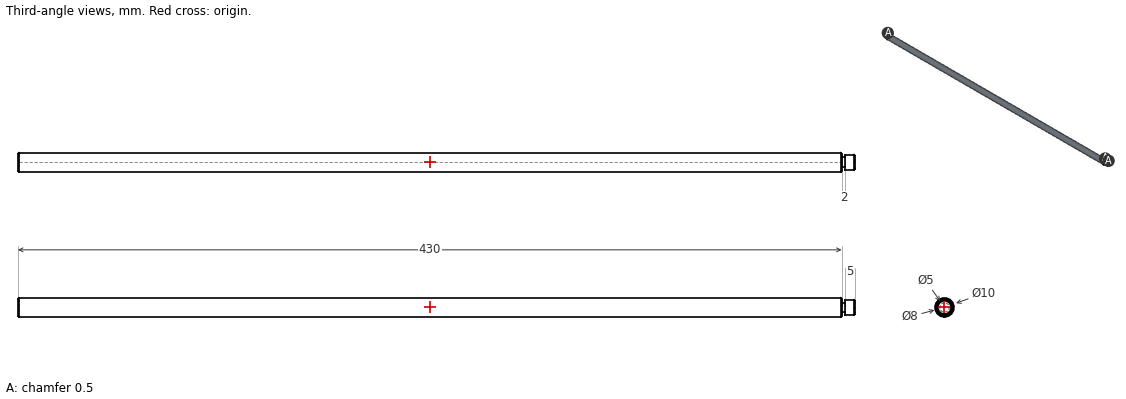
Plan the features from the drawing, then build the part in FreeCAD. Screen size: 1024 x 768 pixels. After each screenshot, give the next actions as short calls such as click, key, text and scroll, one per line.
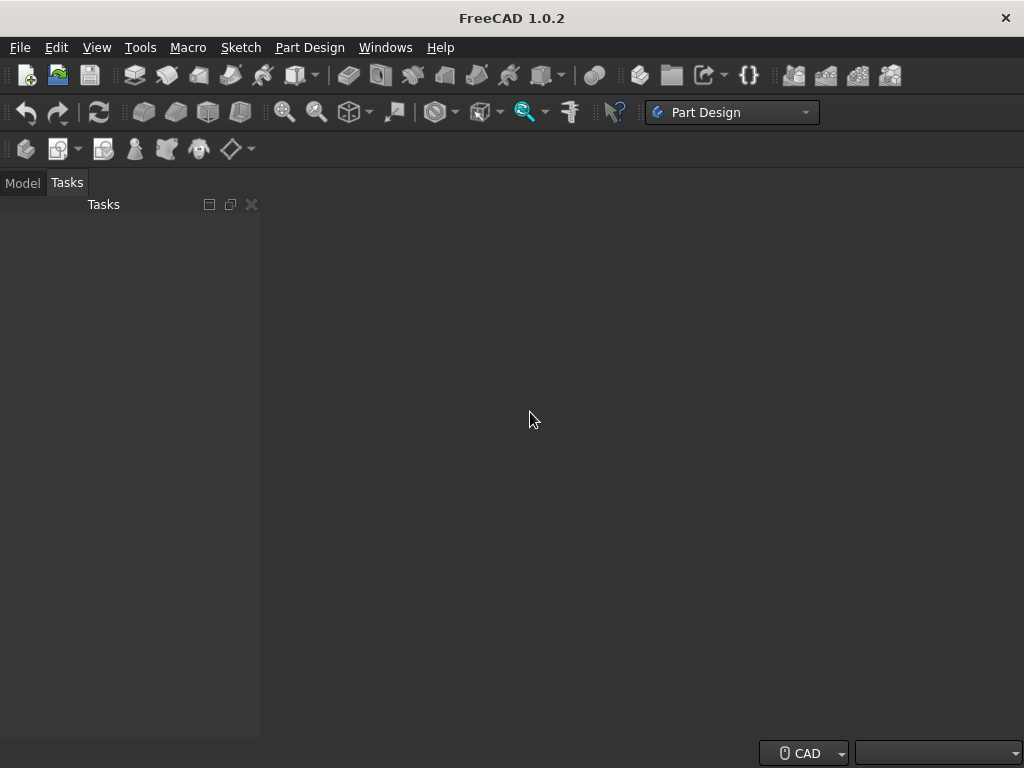
click(26, 76)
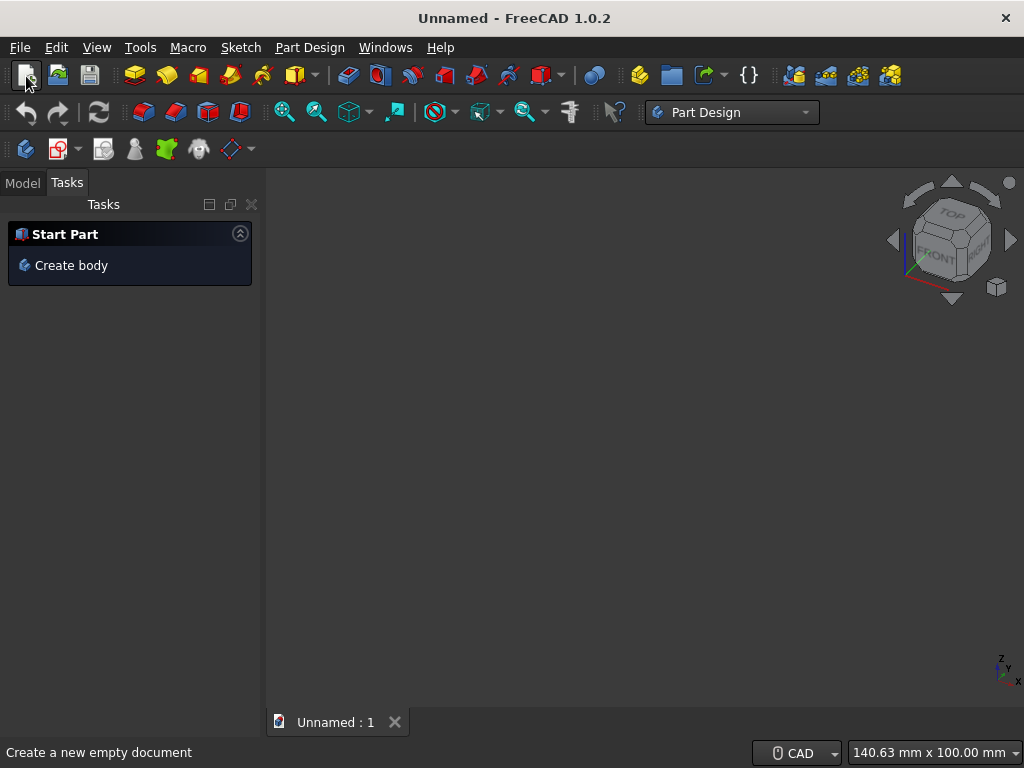
click(58, 150)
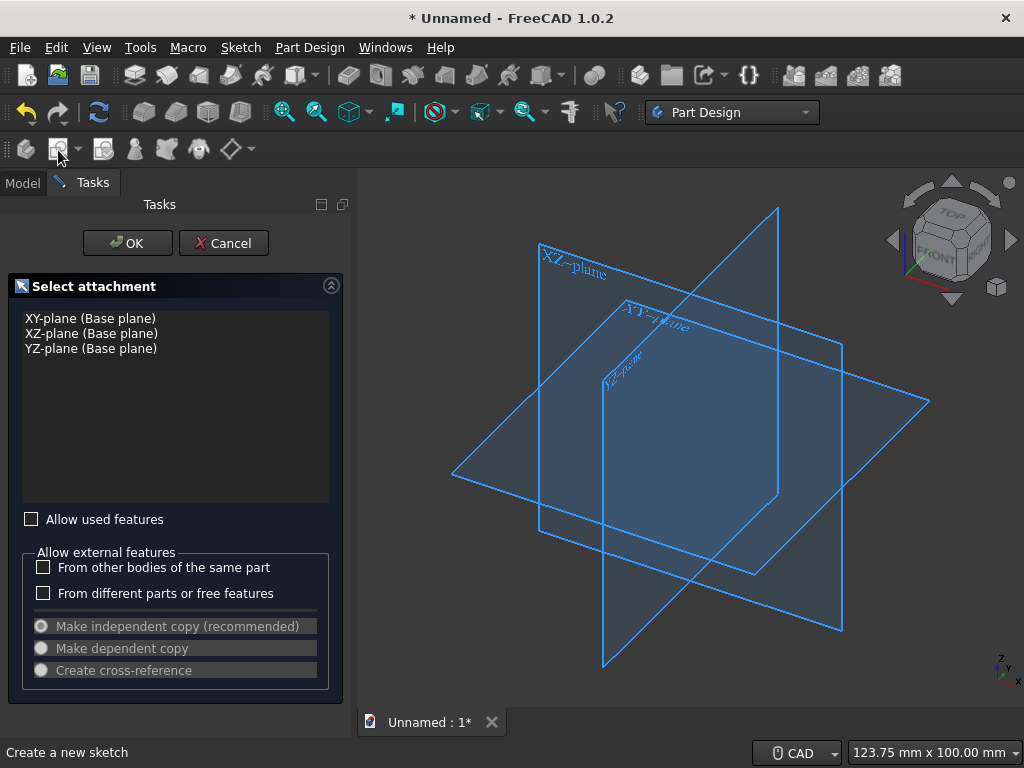
click(82, 348)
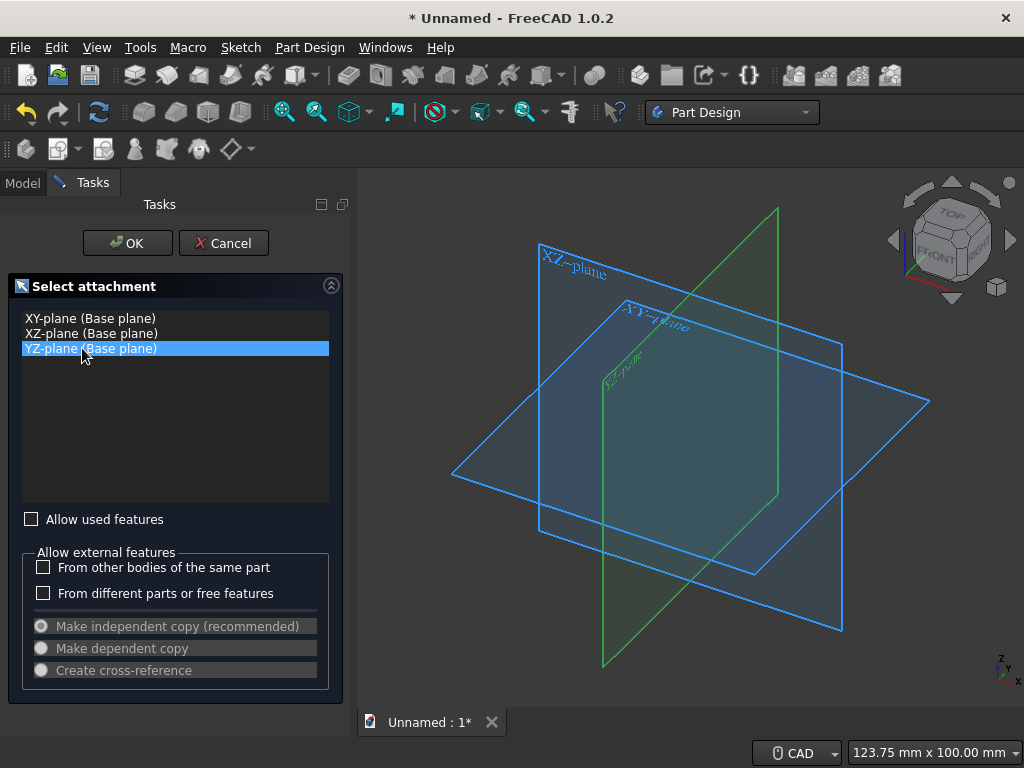
click(128, 243)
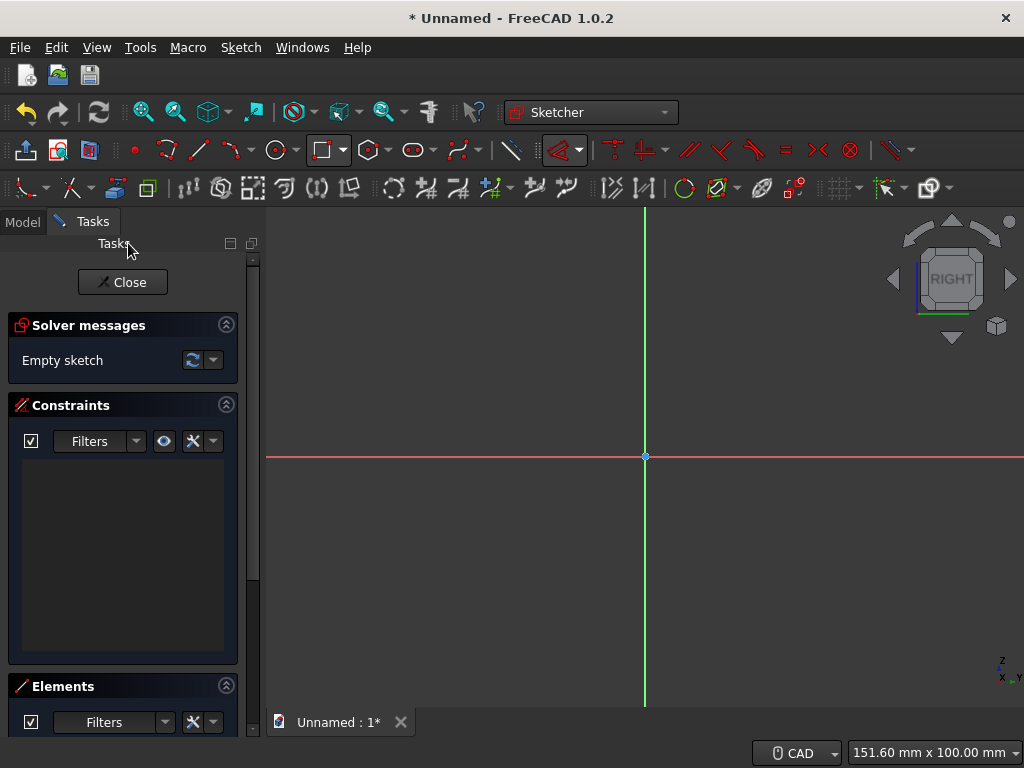
scroll(659, 457, up, 9)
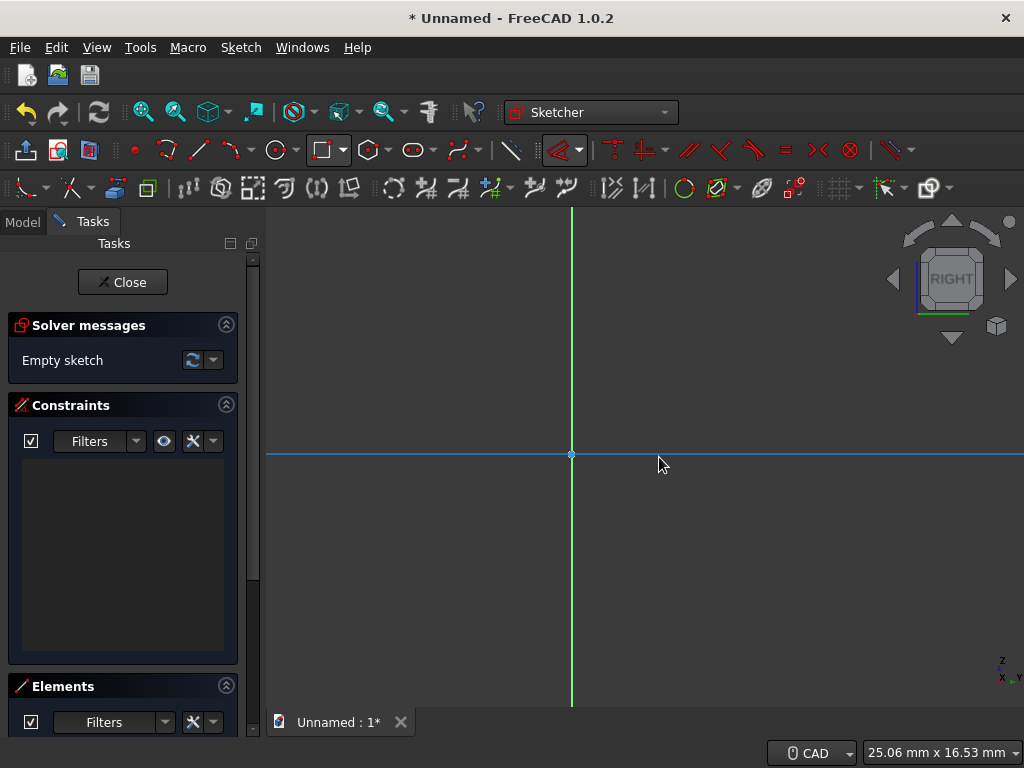
click(276, 150)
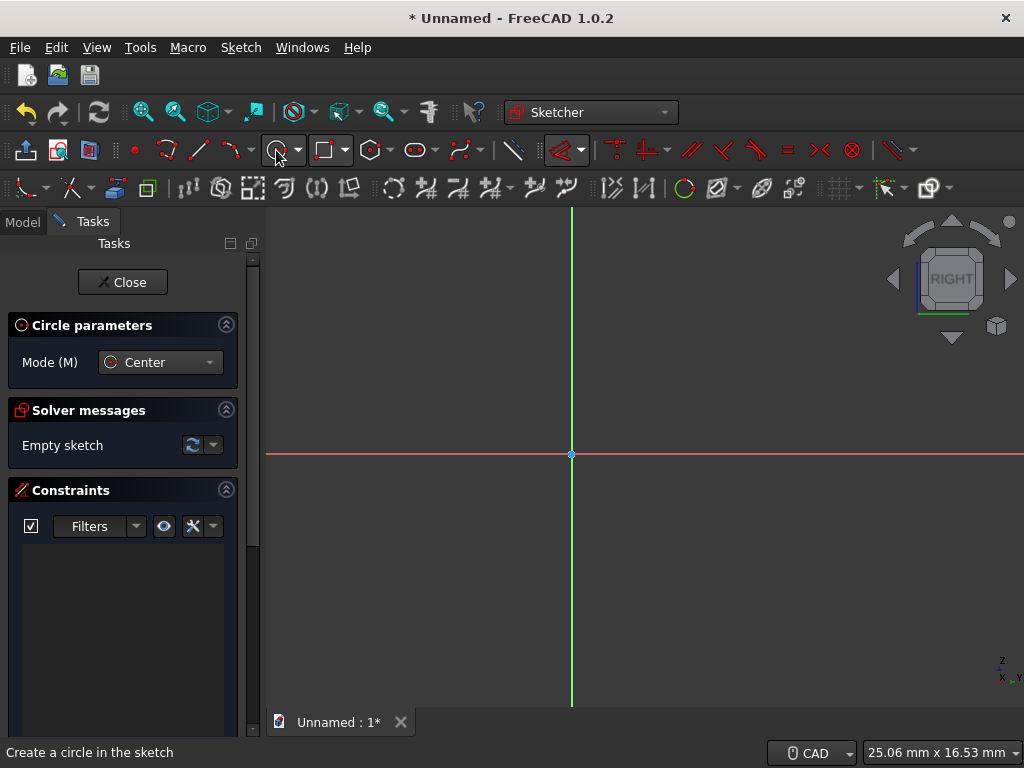
click(572, 454)
move(679, 348)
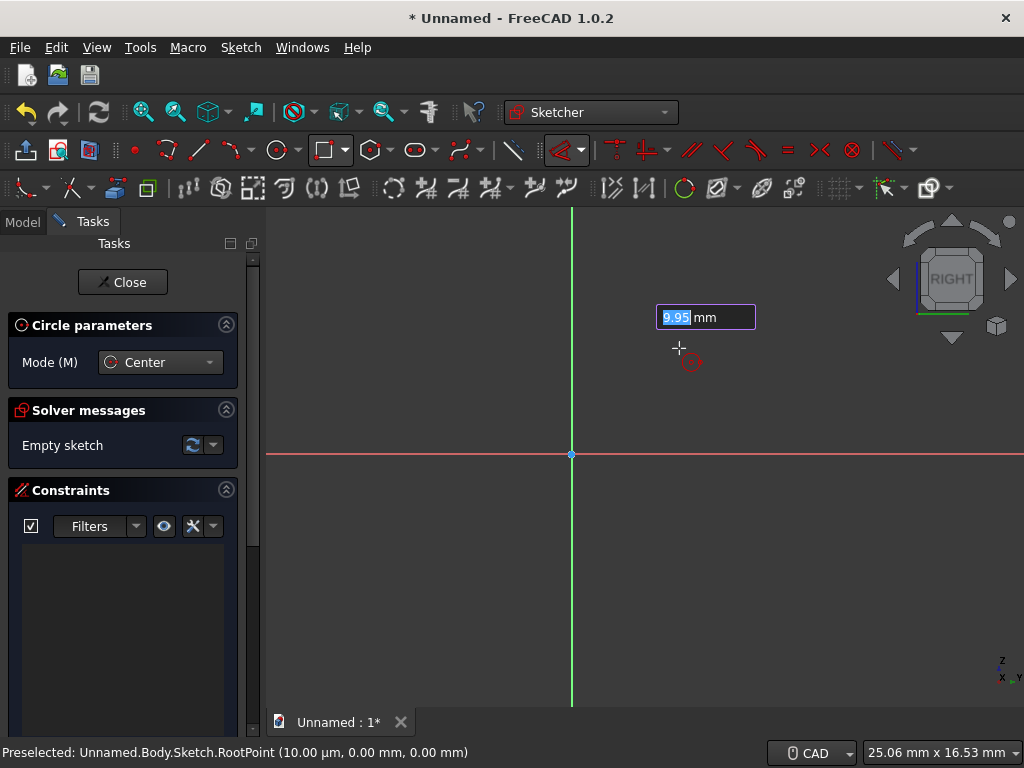
text(10)
key(Return)
key(Escape)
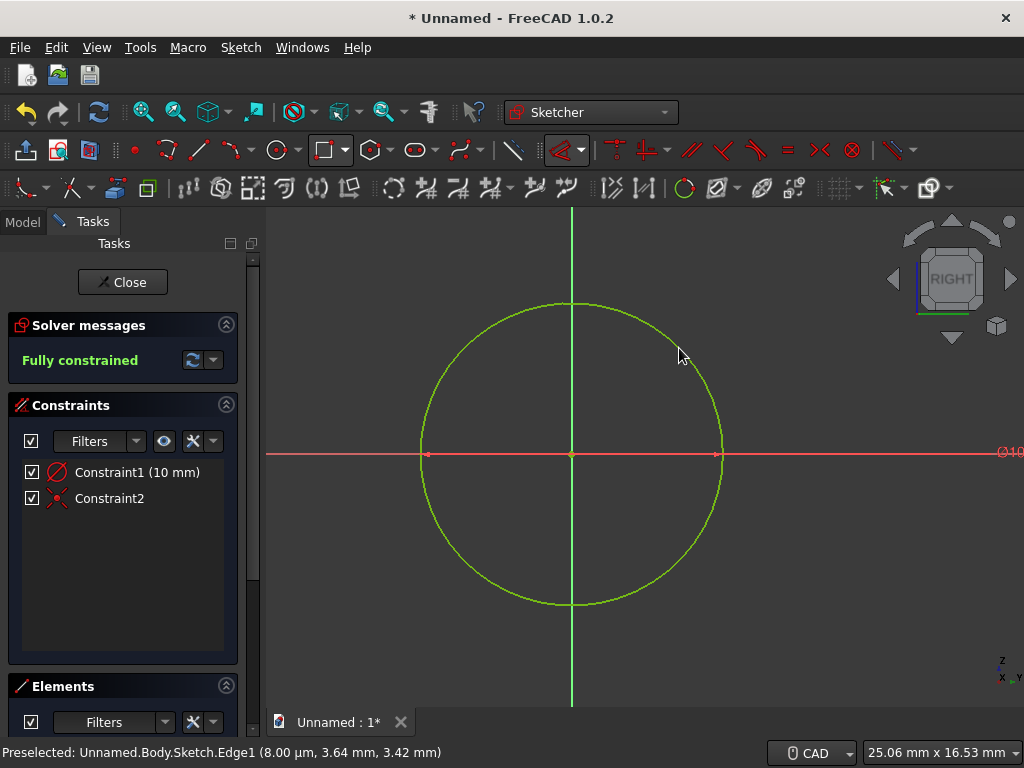
click(123, 282)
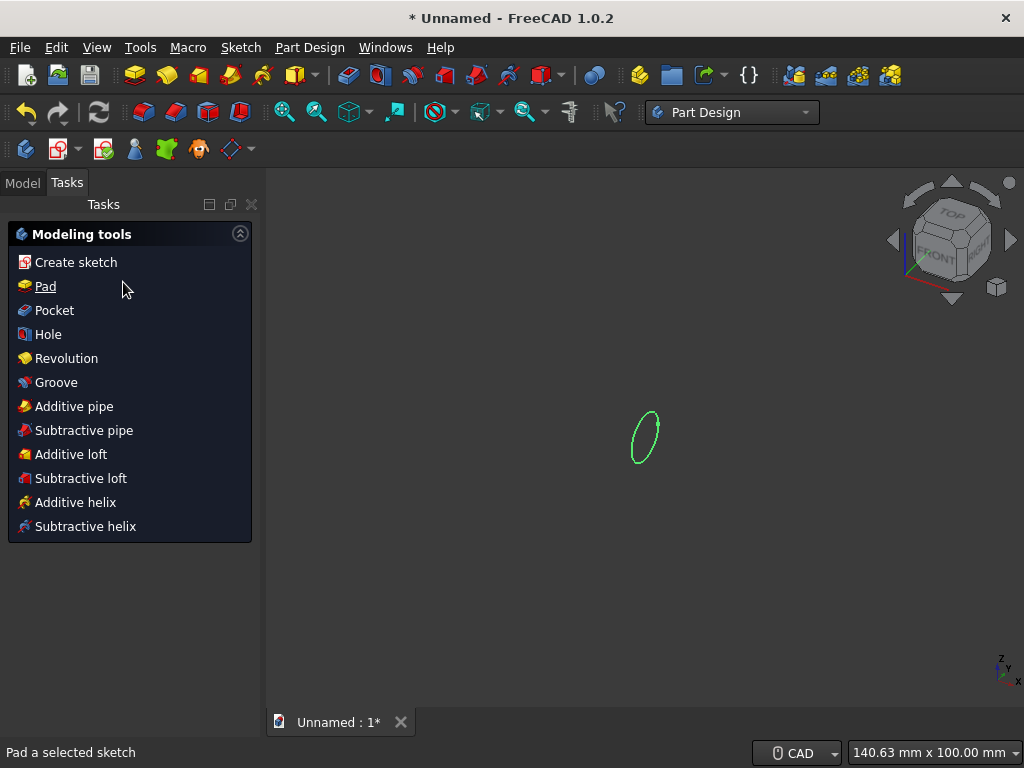
click(136, 76)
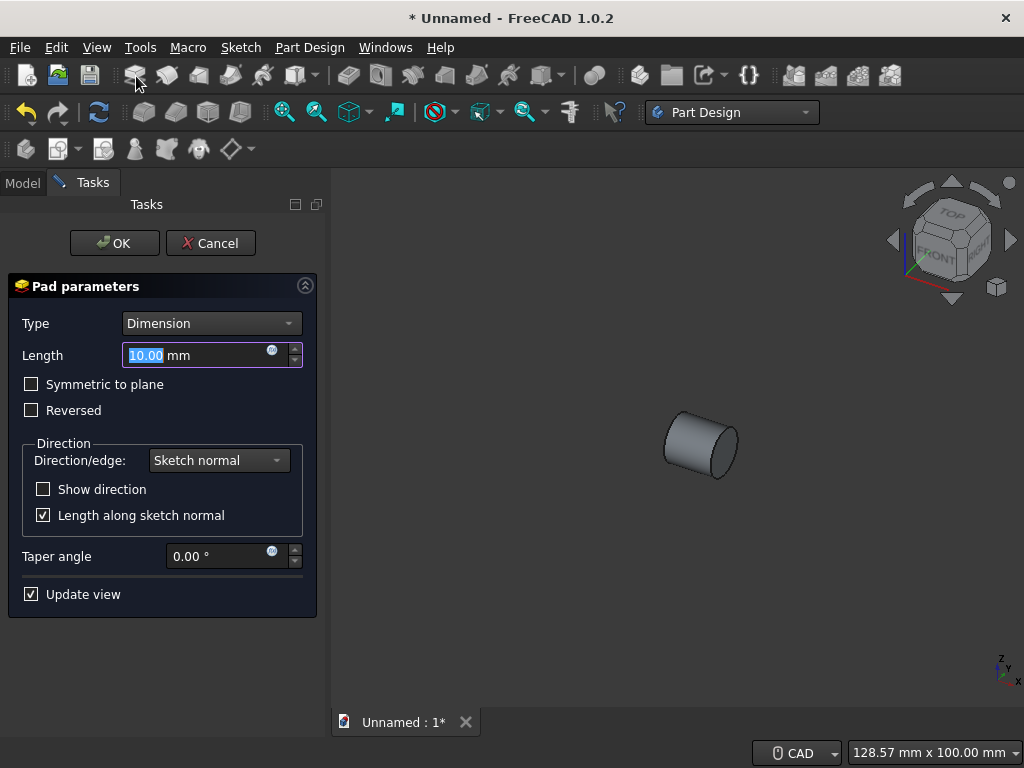
text(430)
key(Tab)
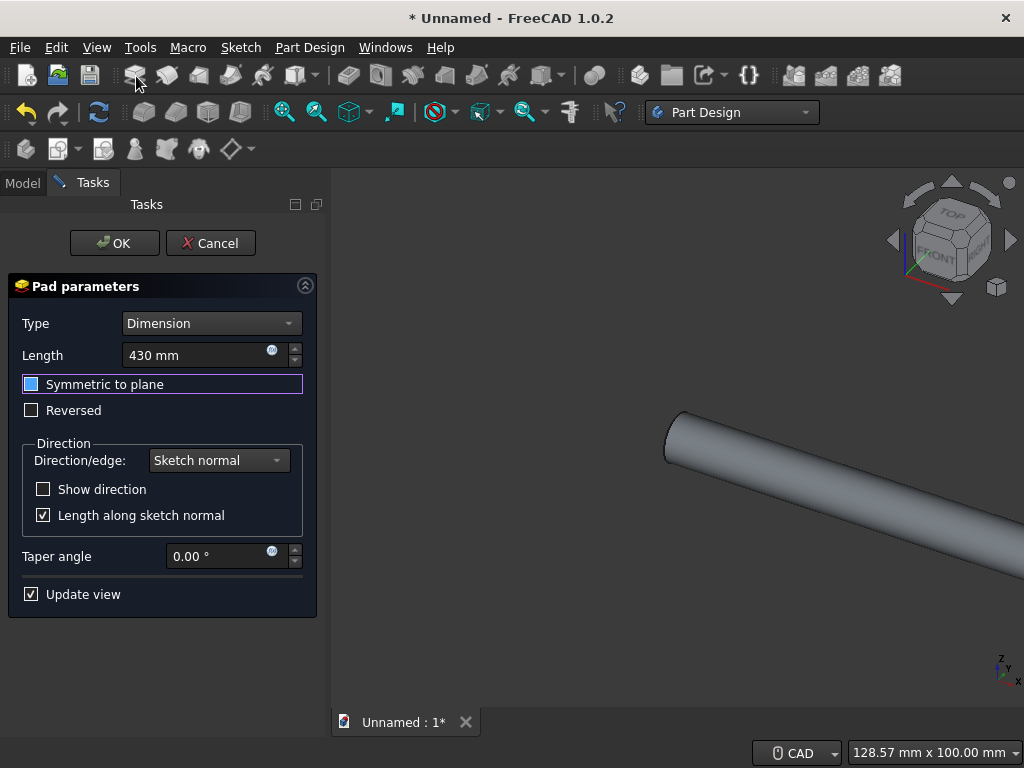
click(30, 384)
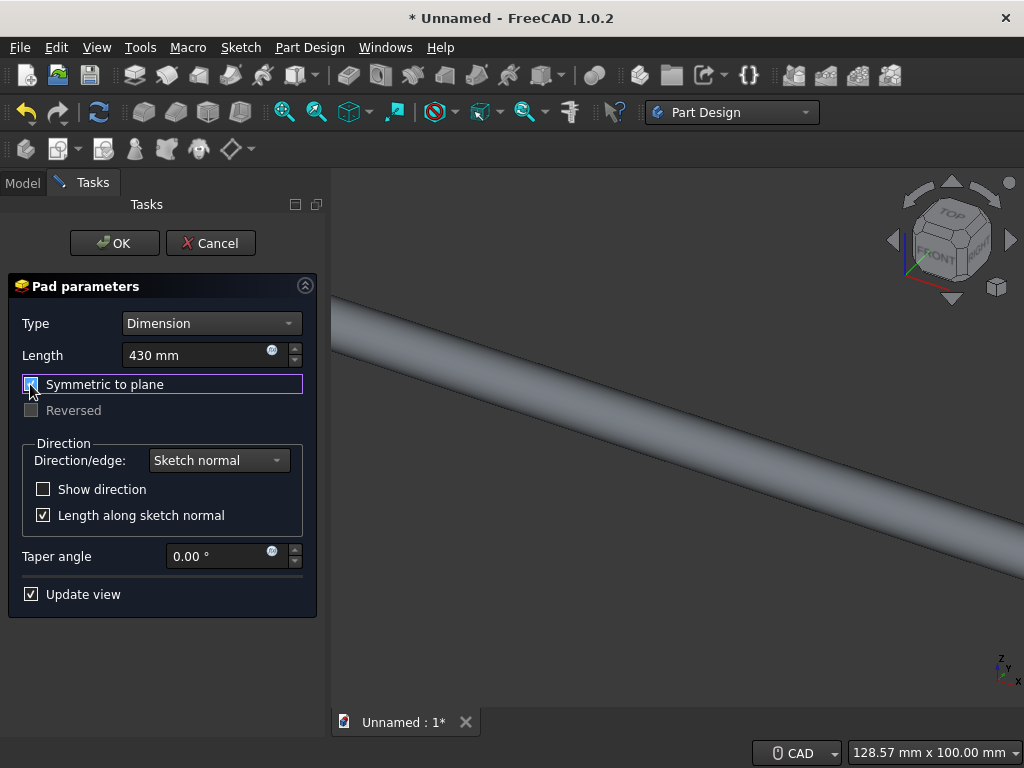
click(115, 243)